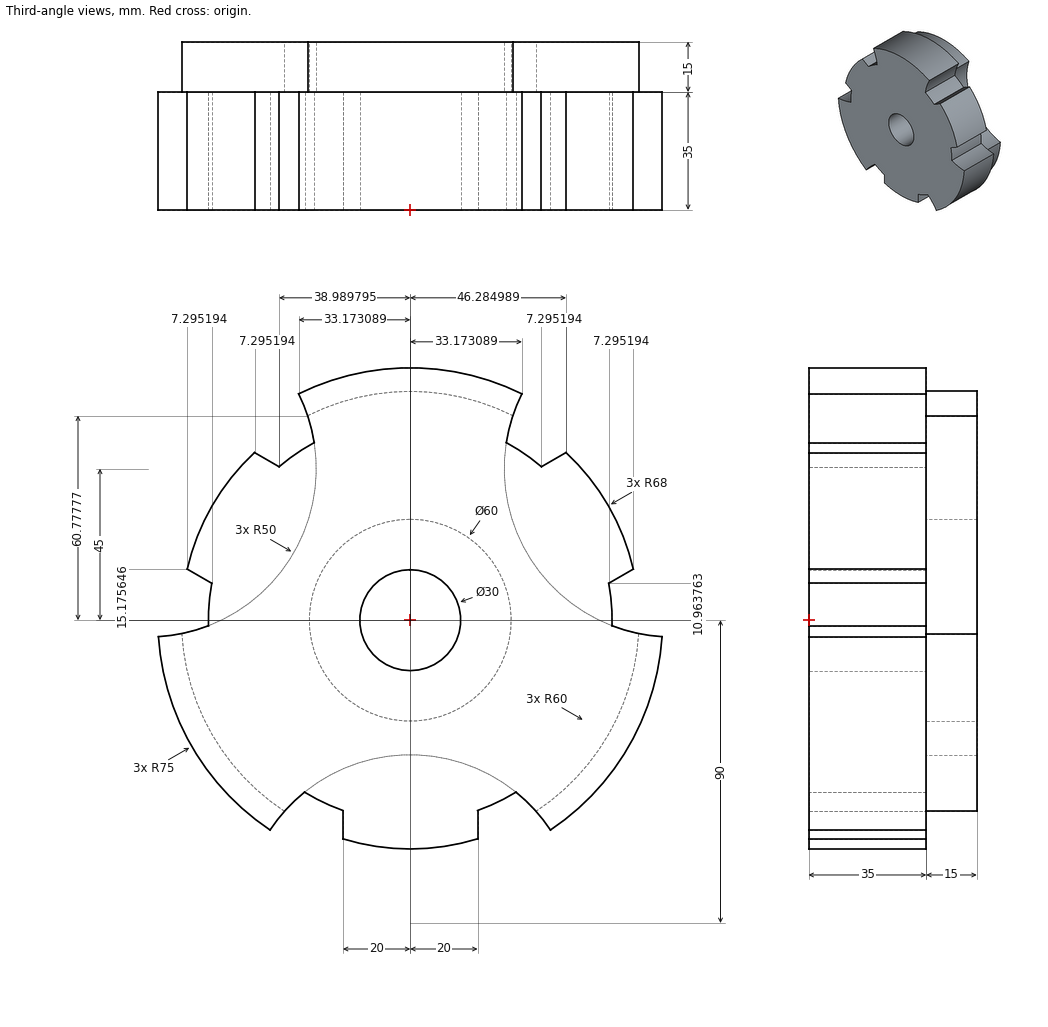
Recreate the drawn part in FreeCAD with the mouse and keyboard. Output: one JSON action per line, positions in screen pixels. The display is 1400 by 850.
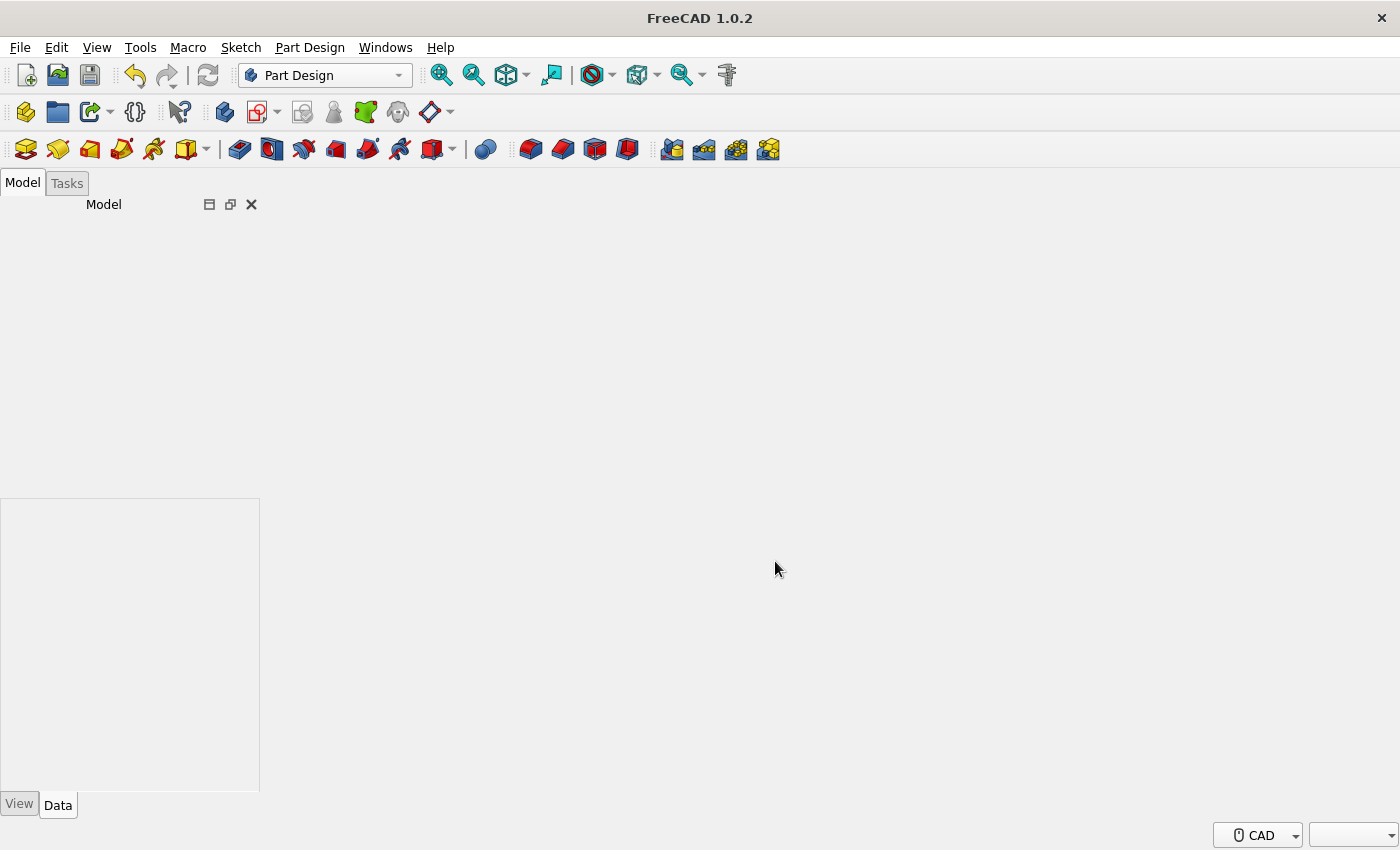
{"action": "left_click", "coordinate": [26, 76]}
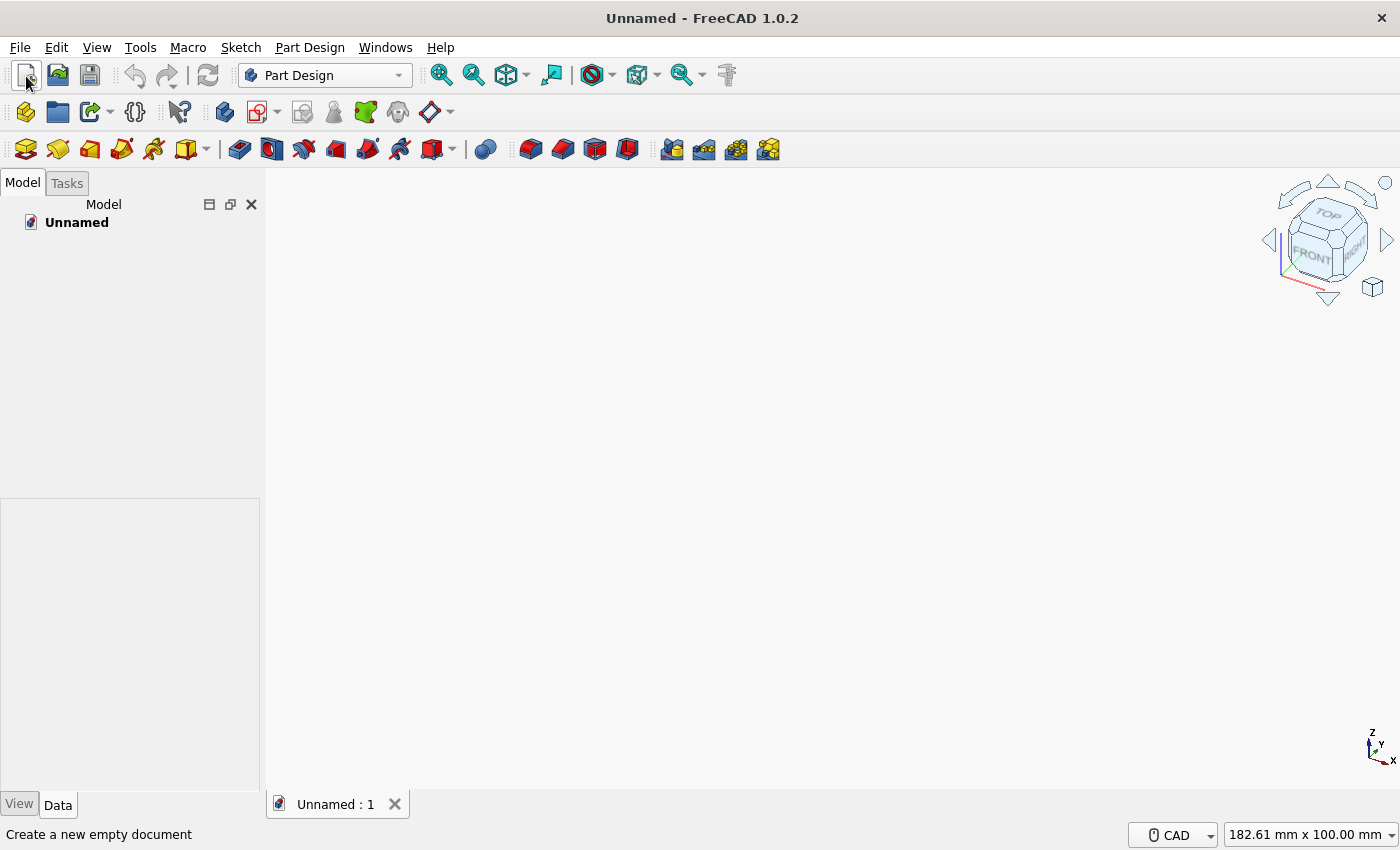
{"action": "left_click", "coordinate": [258, 112]}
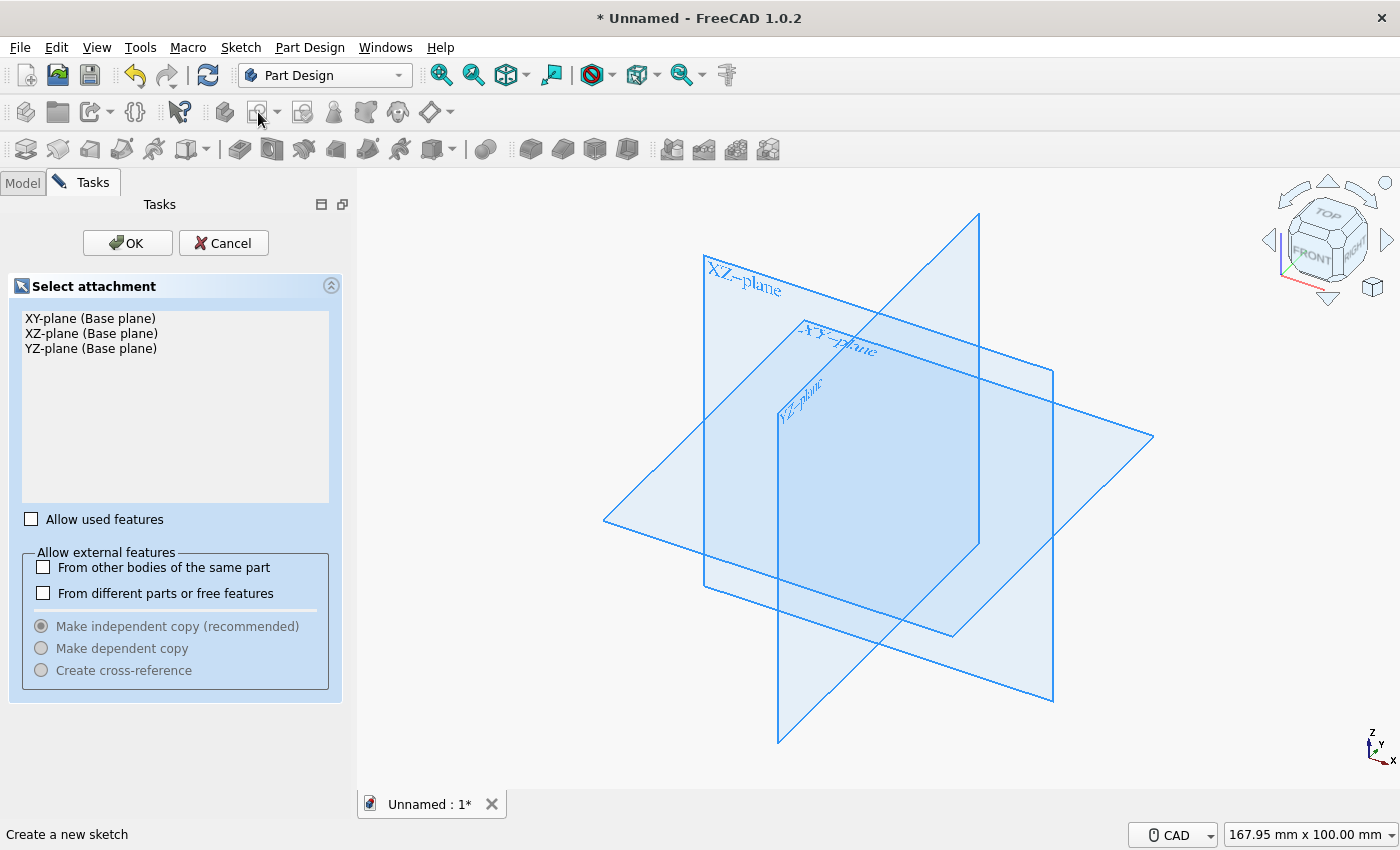
{"action": "left_click", "coordinate": [82, 334]}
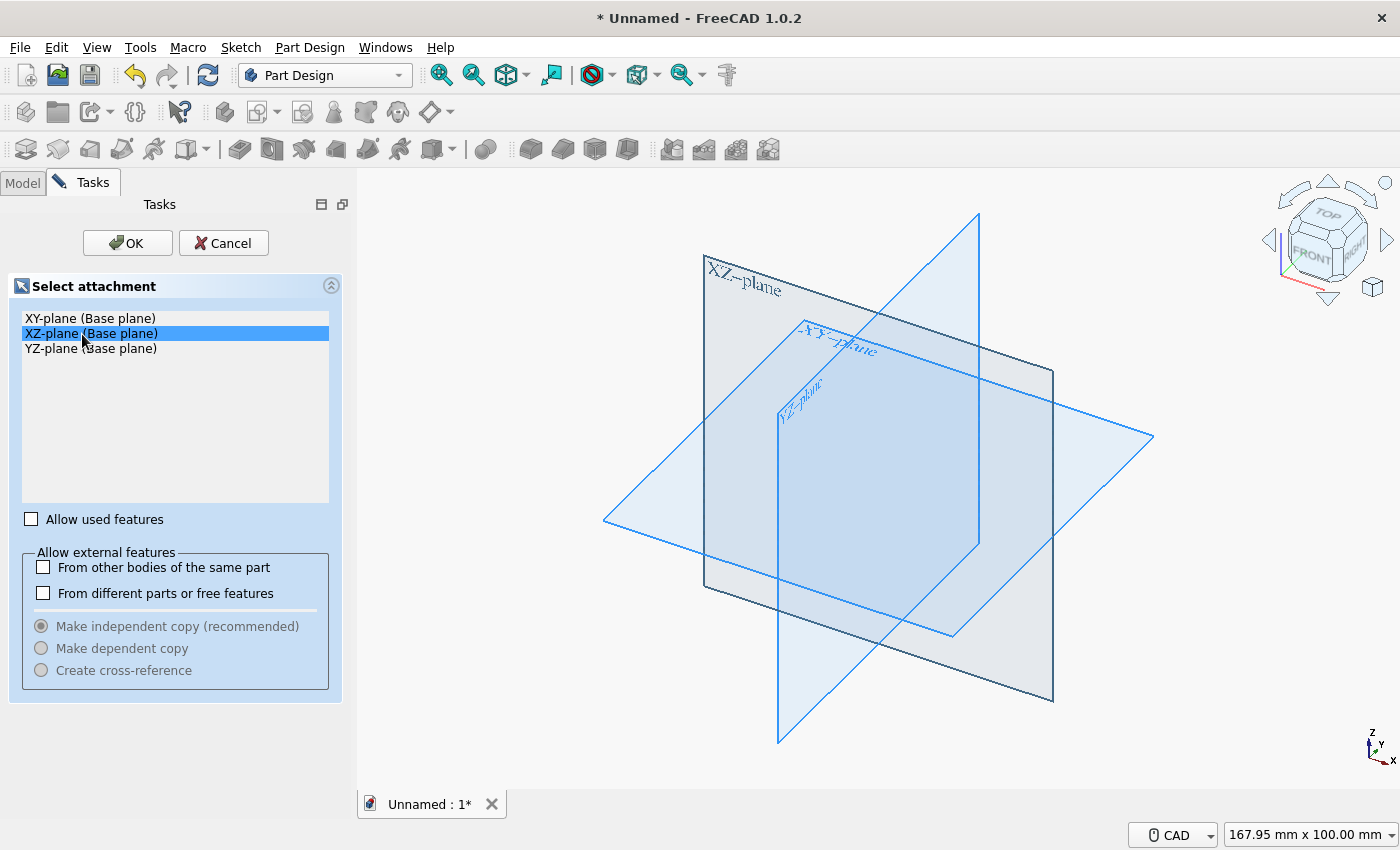
{"action": "left_click", "coordinate": [128, 243]}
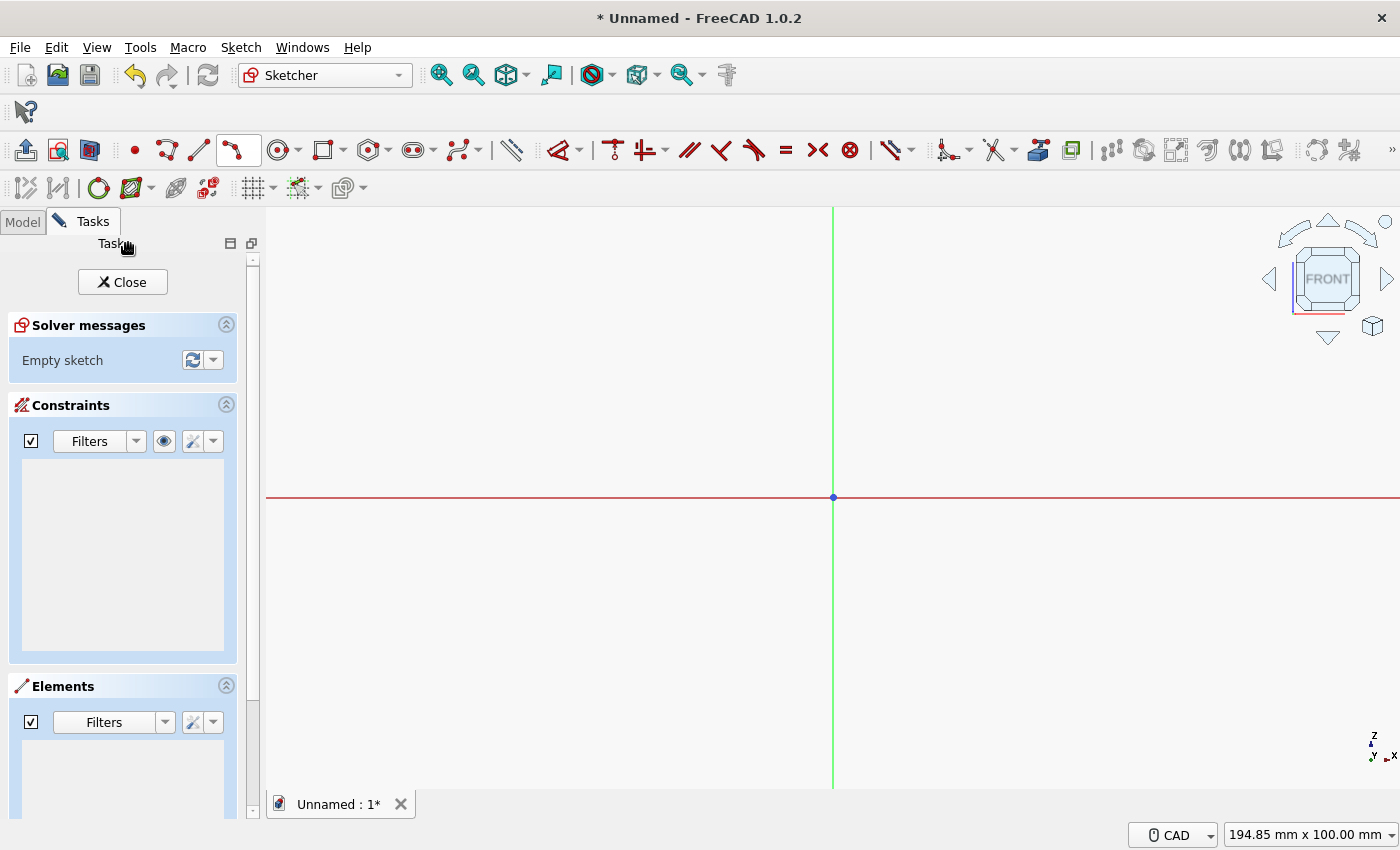
{"action": "scroll", "coordinate": [709, 528], "scroll_direction": "down", "scroll_amount": 4}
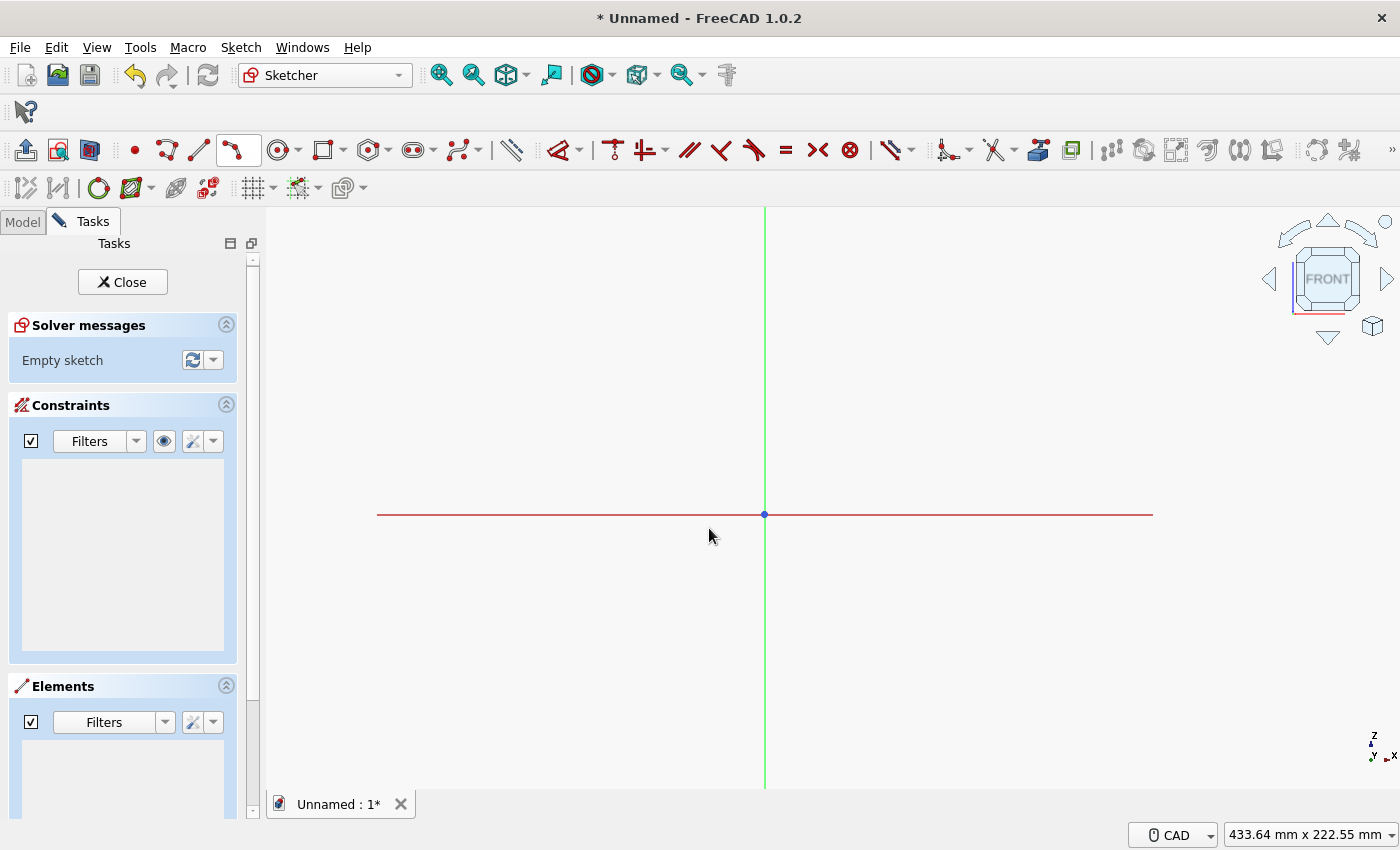
{"action": "key", "text": "g 3 a"}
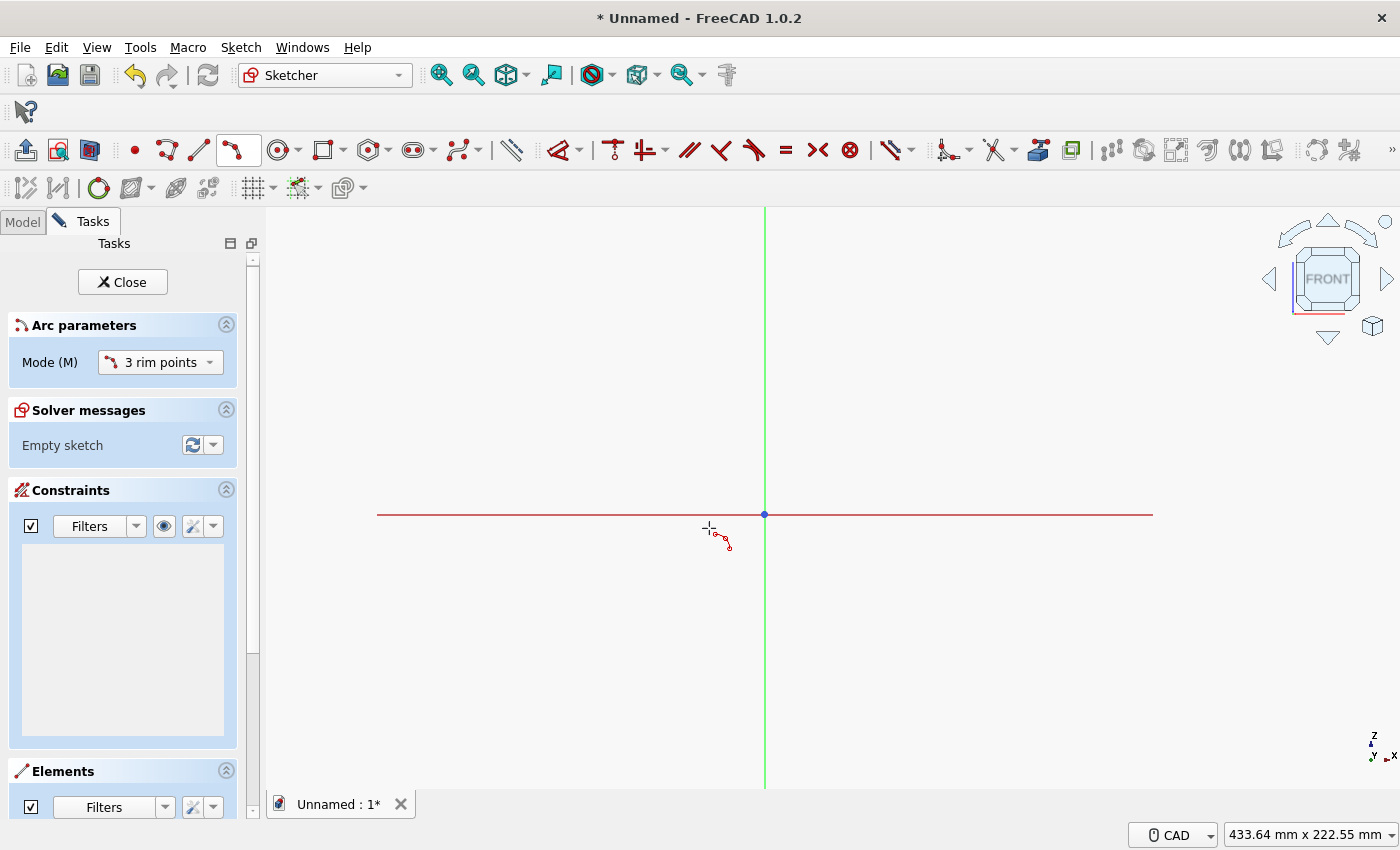
{"action": "left_click", "coordinate": [656, 678]}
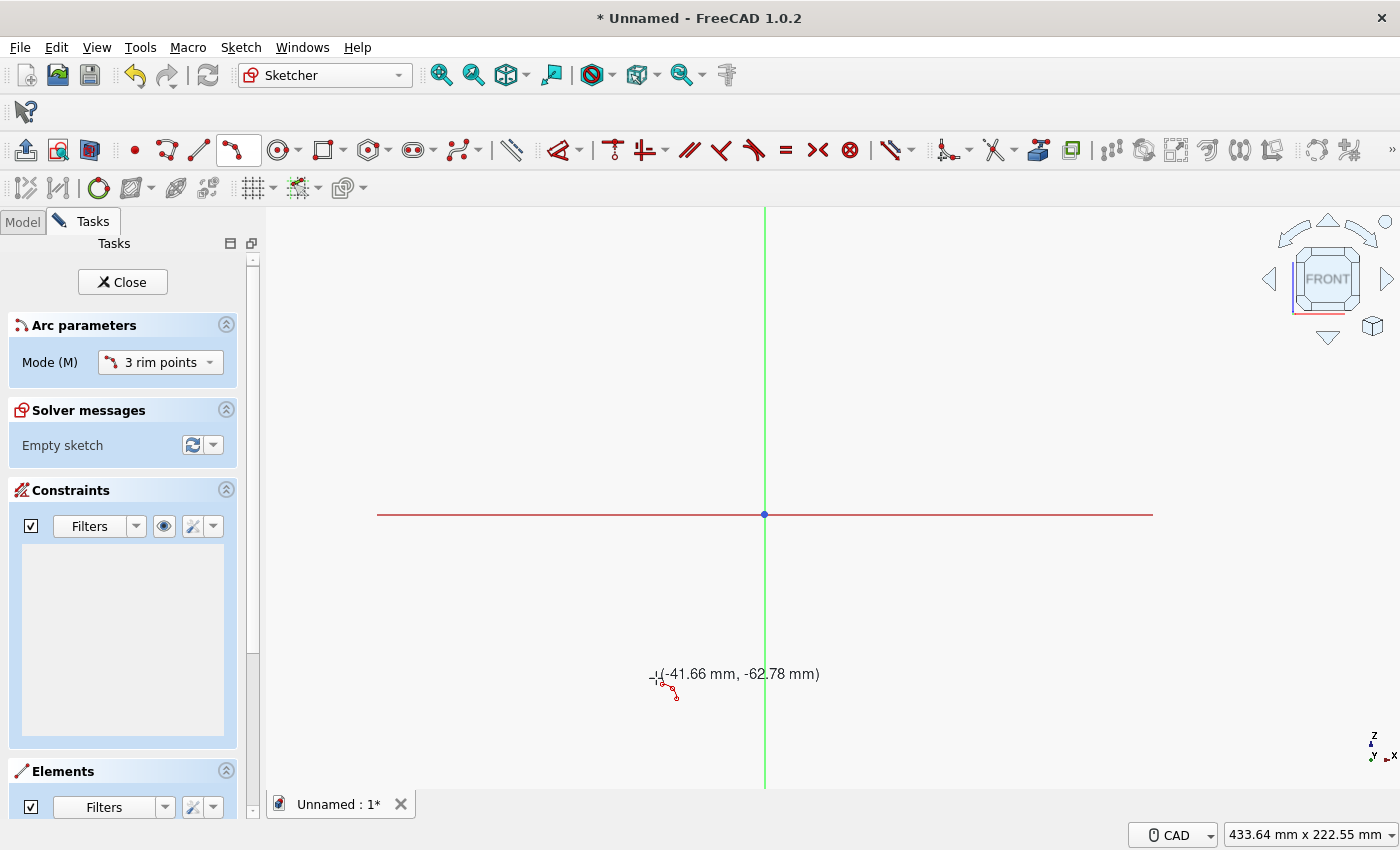
{"action": "scroll", "coordinate": [569, 528], "scroll_direction": "up", "scroll_amount": 2}